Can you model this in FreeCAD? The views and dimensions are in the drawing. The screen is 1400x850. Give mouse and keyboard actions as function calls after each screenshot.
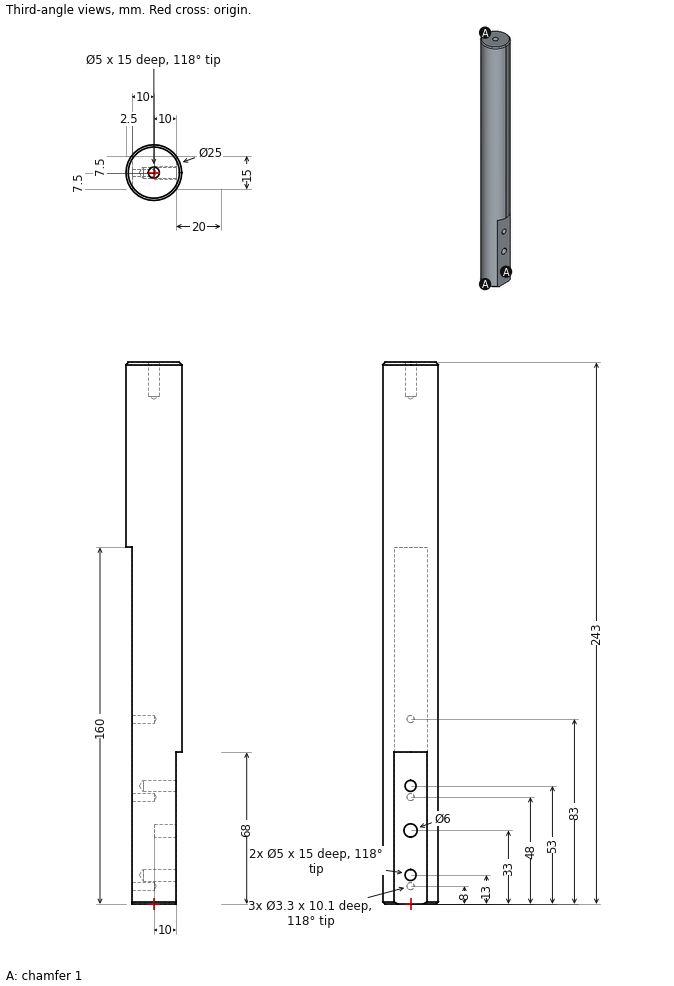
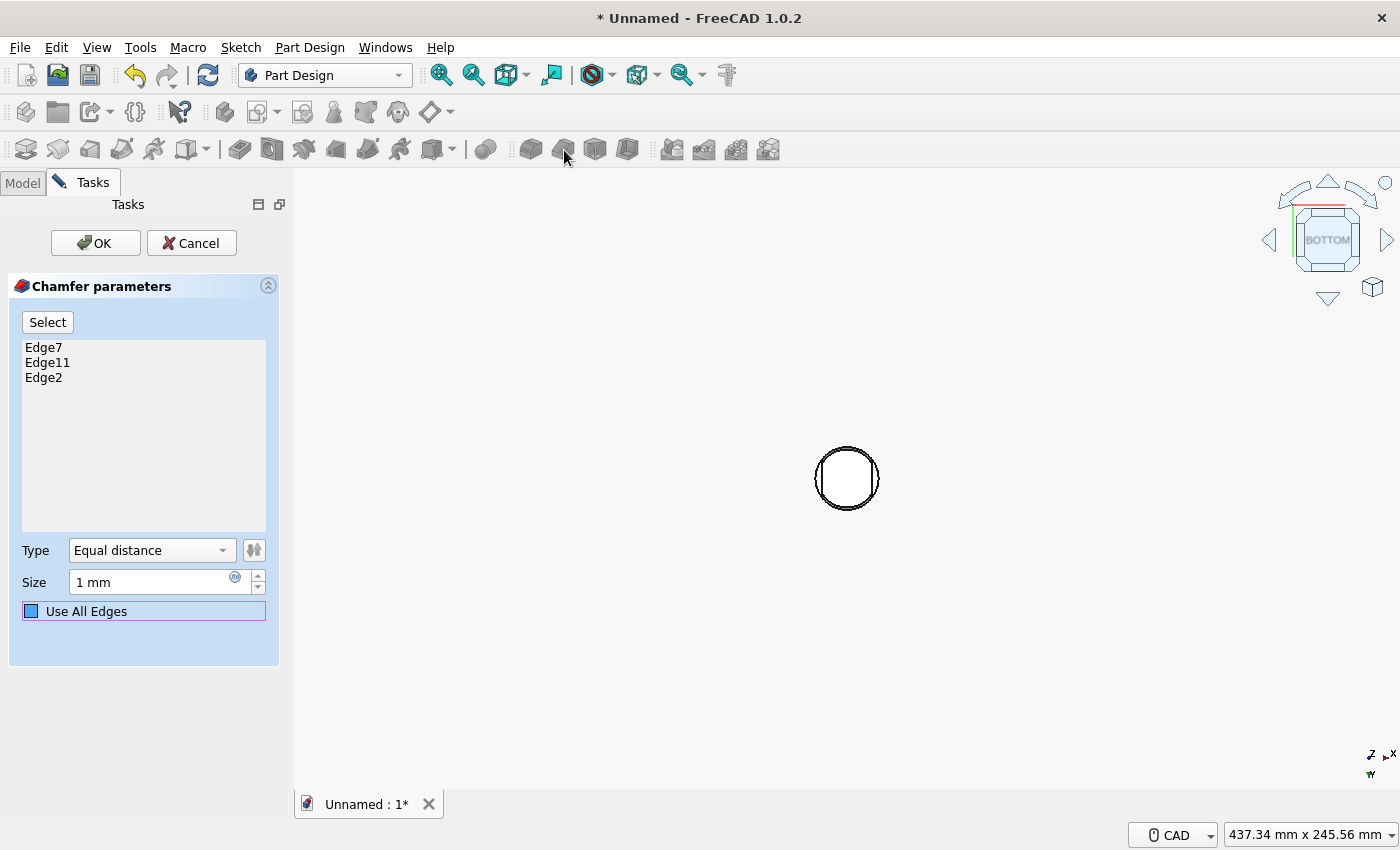
click(96, 243)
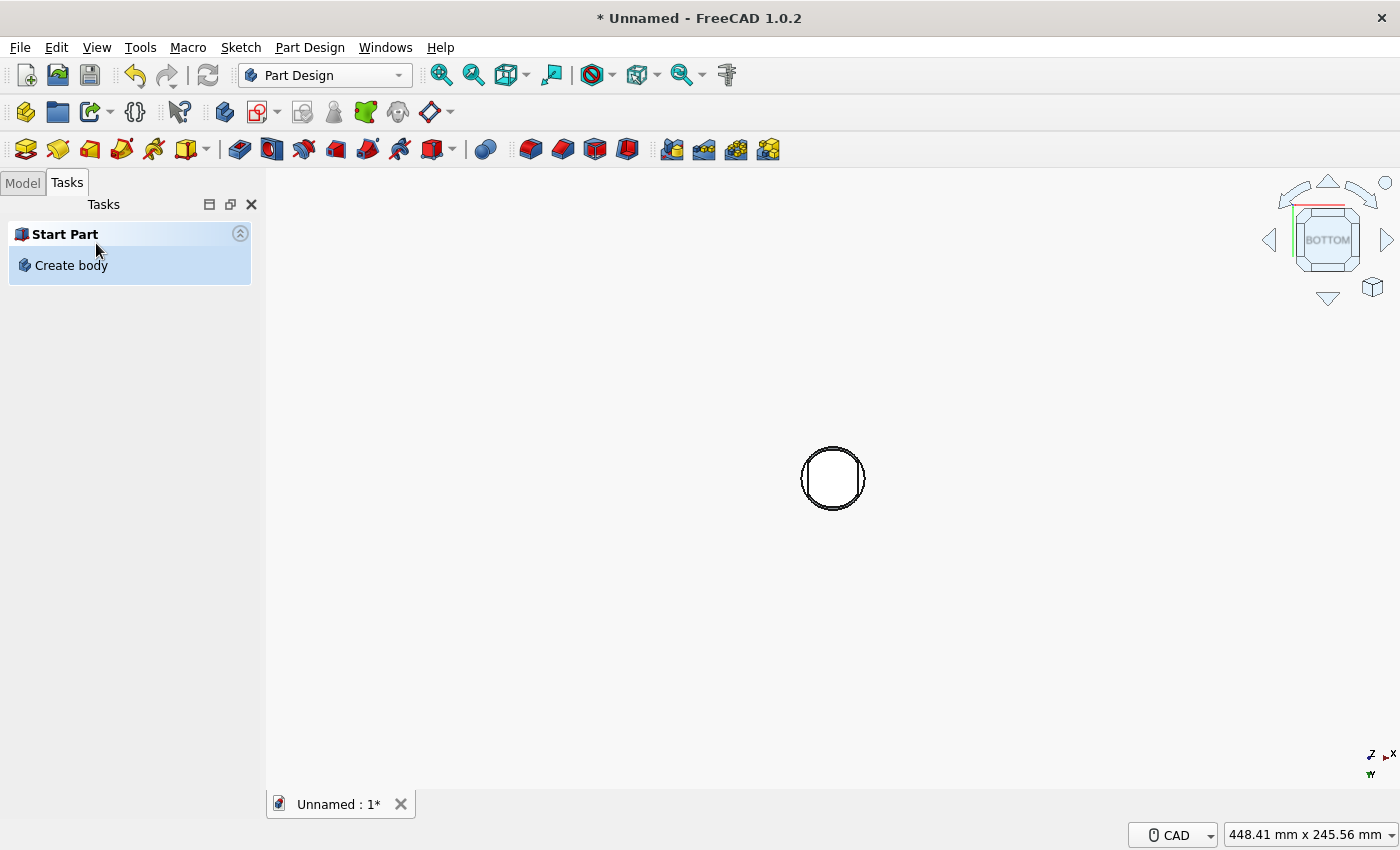
key(0)